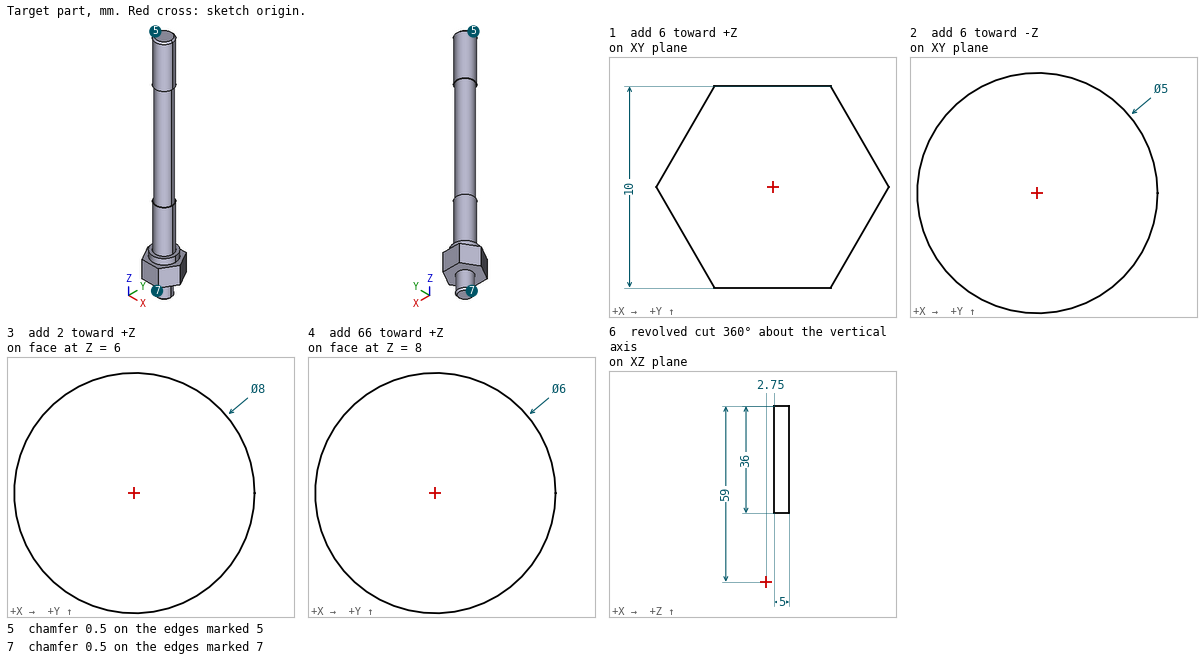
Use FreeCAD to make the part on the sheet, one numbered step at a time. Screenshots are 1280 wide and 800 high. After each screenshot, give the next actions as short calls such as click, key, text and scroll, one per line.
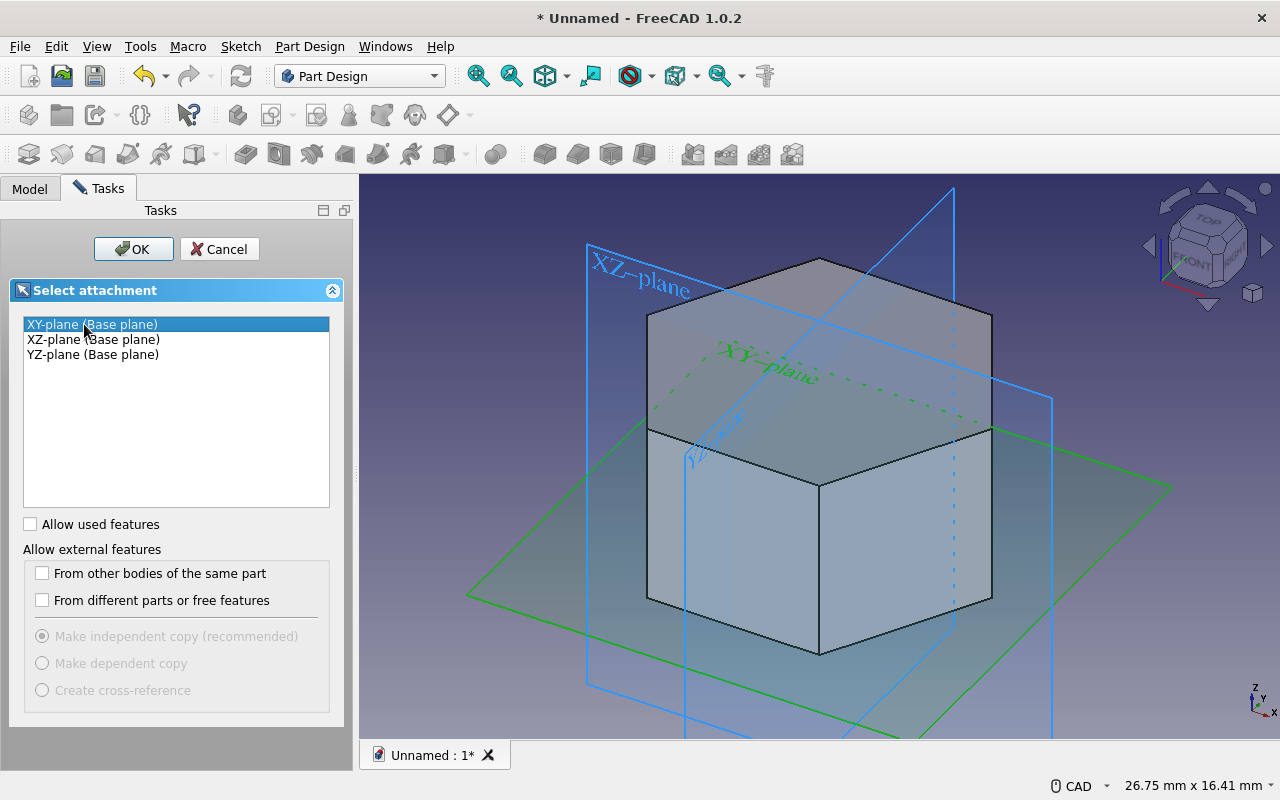
click(134, 249)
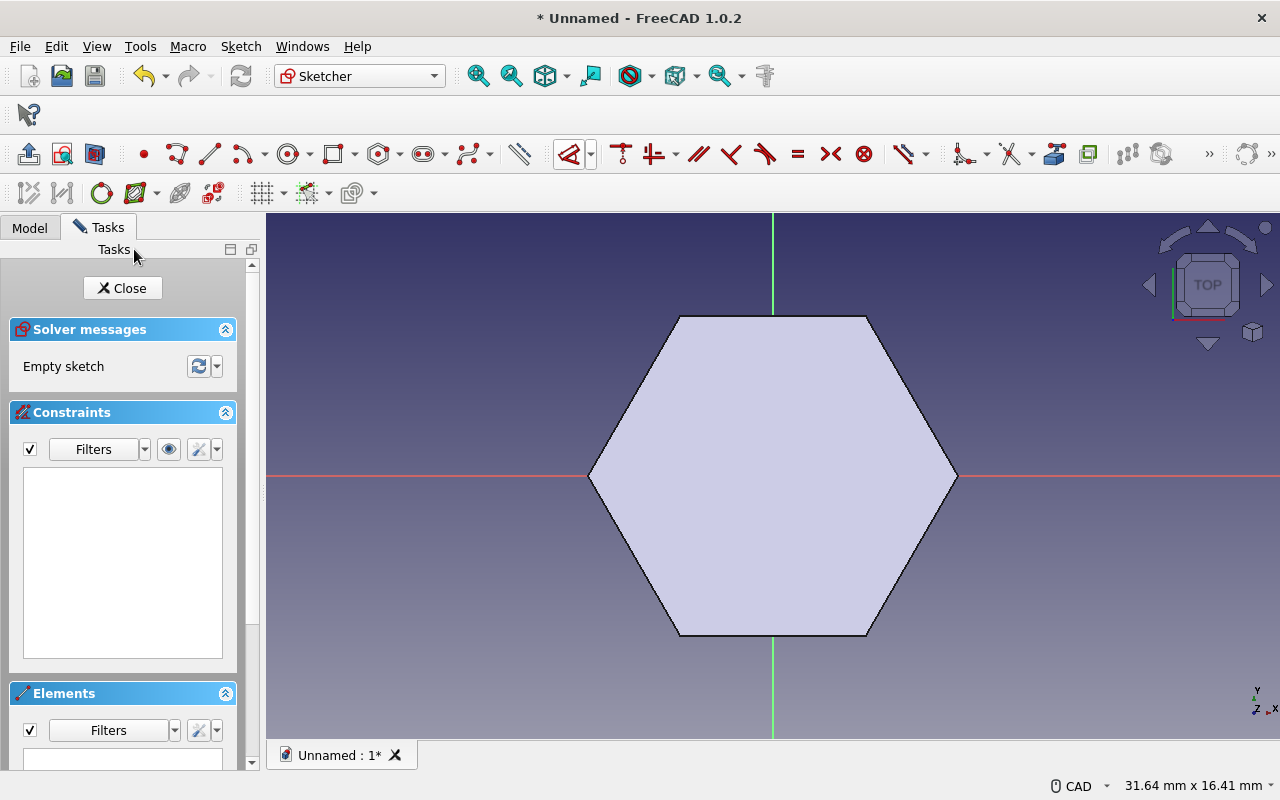
click(95, 154)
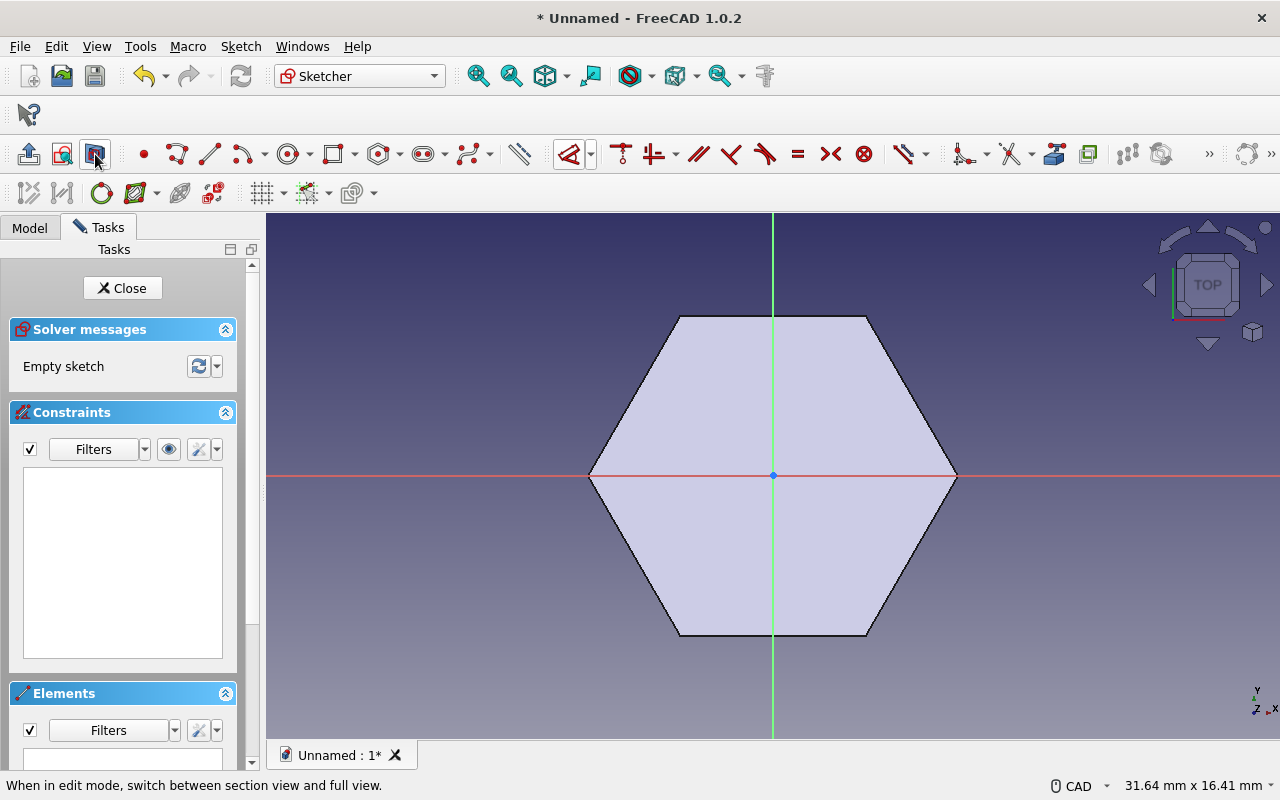
scroll(829, 476, up, 4)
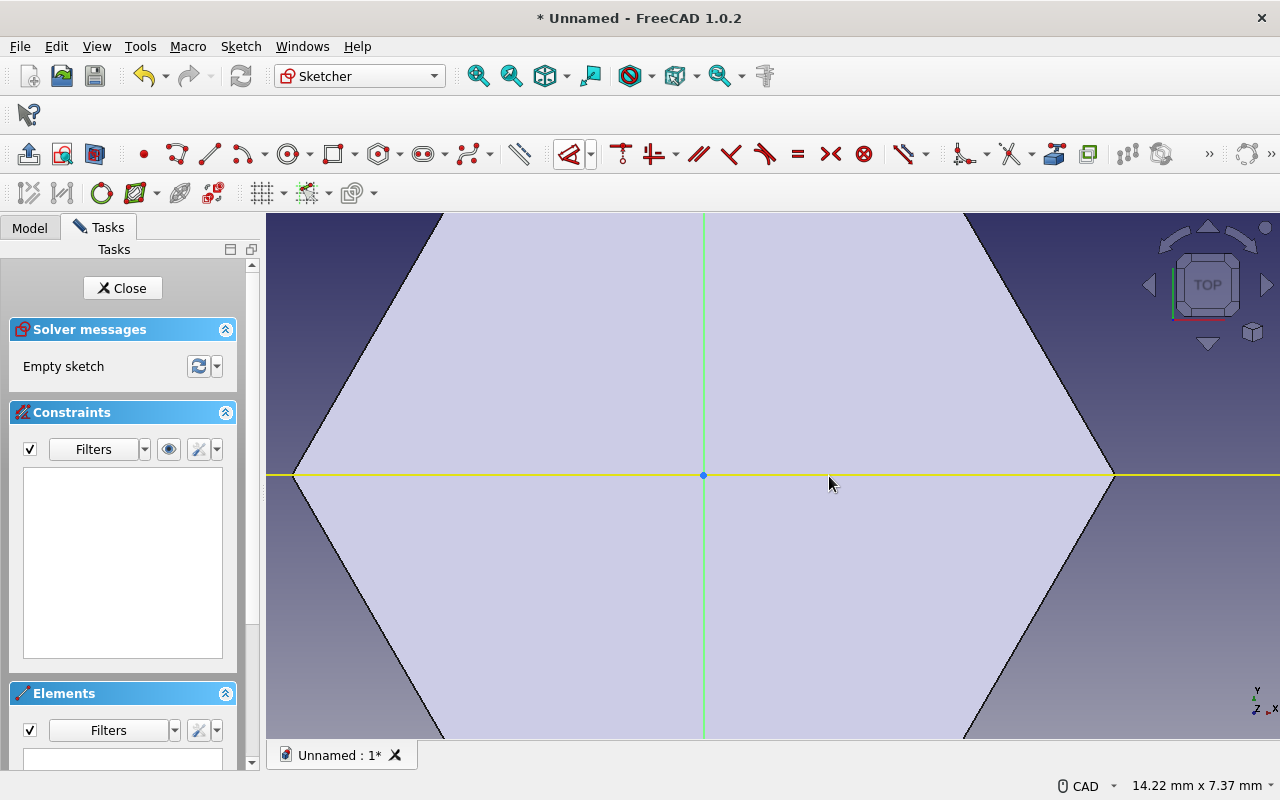
click(288, 154)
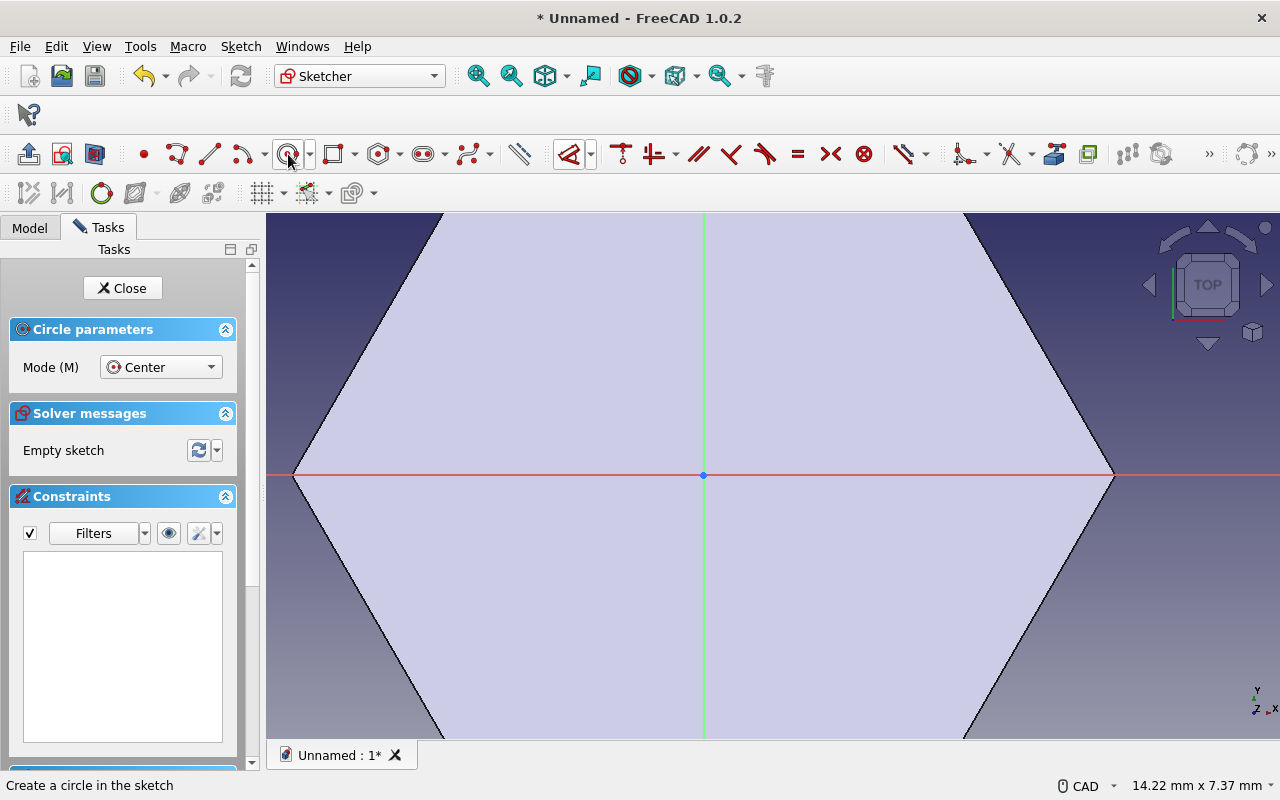
click(704, 475)
click(830, 349)
key(Escape)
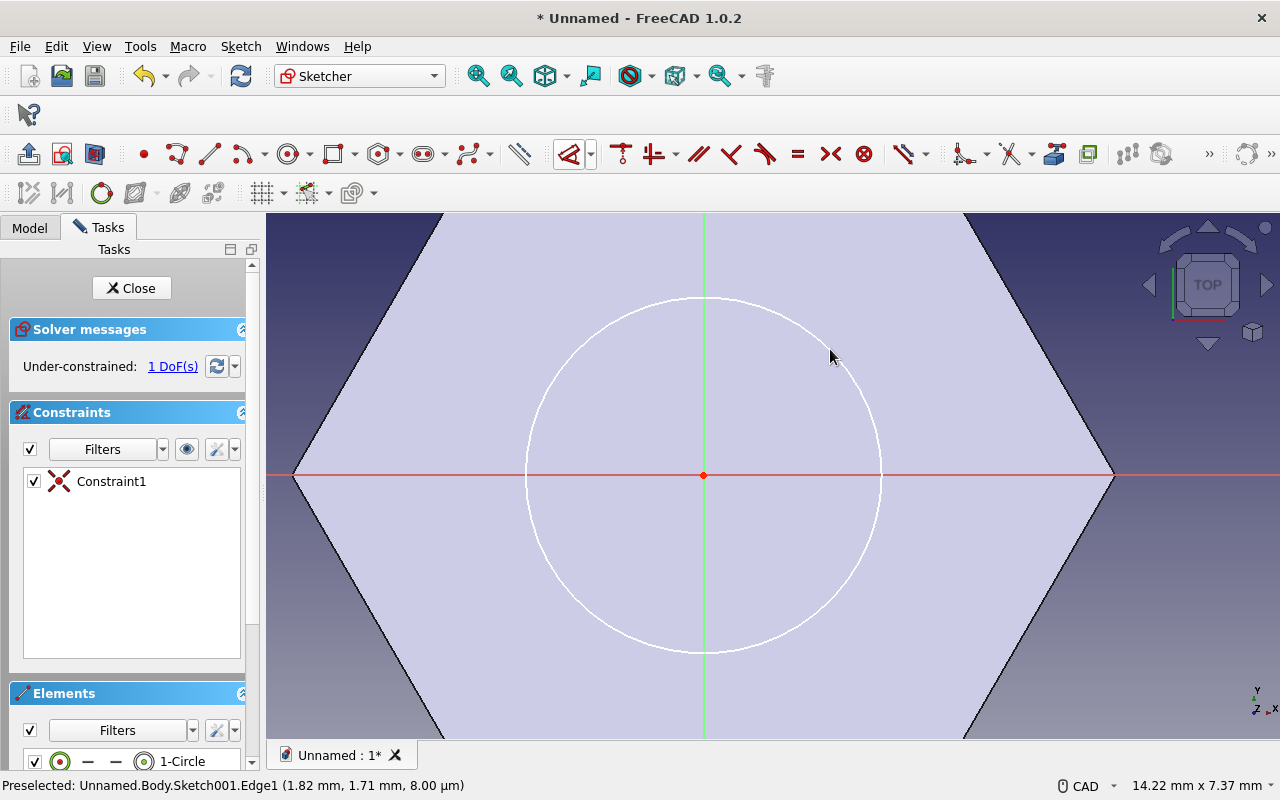
click(829, 349)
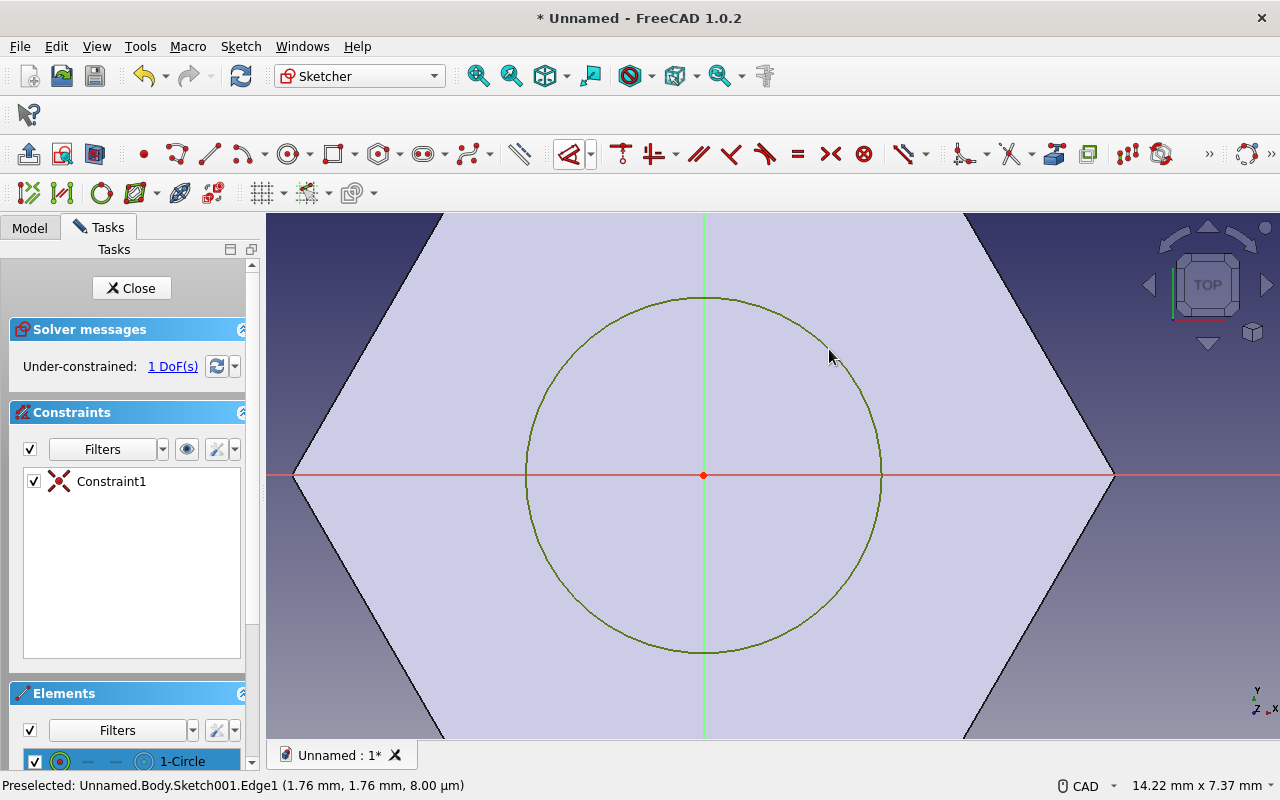
key(k)
key(o)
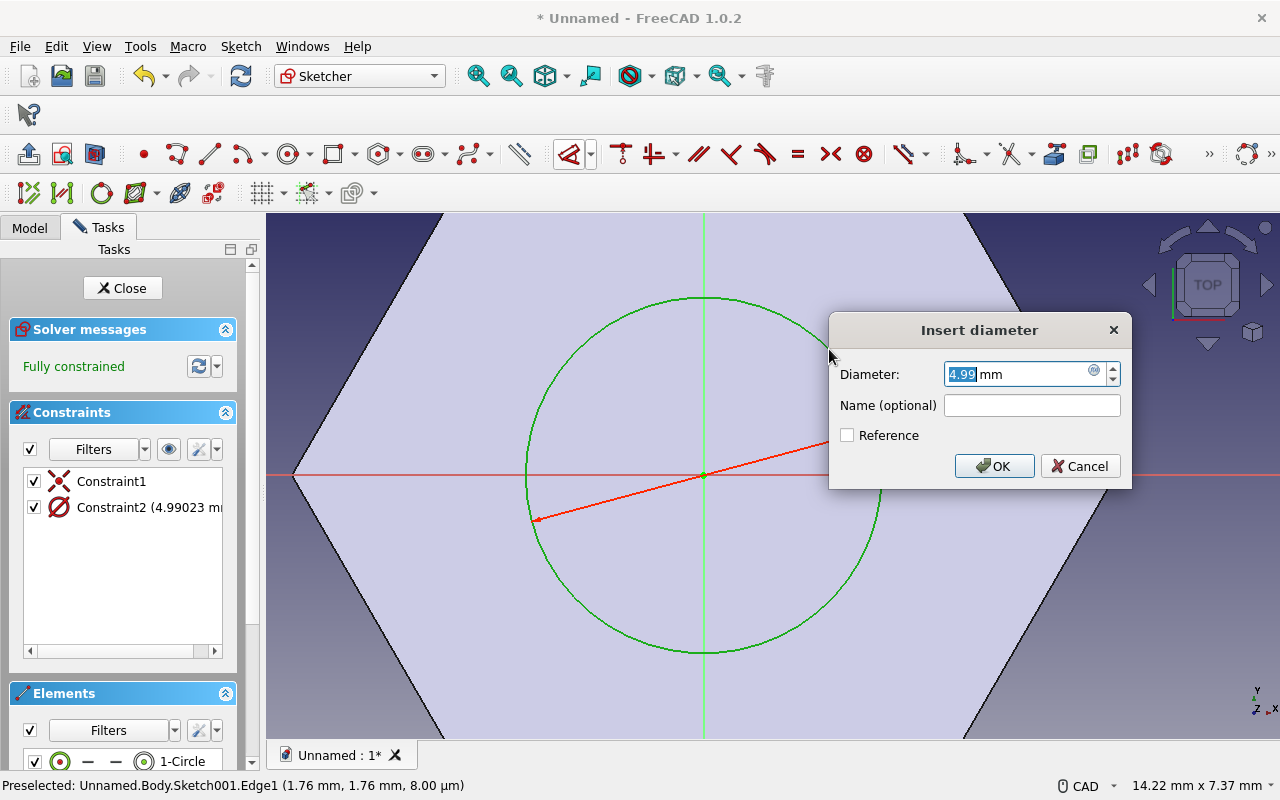
text(5)
key(Return)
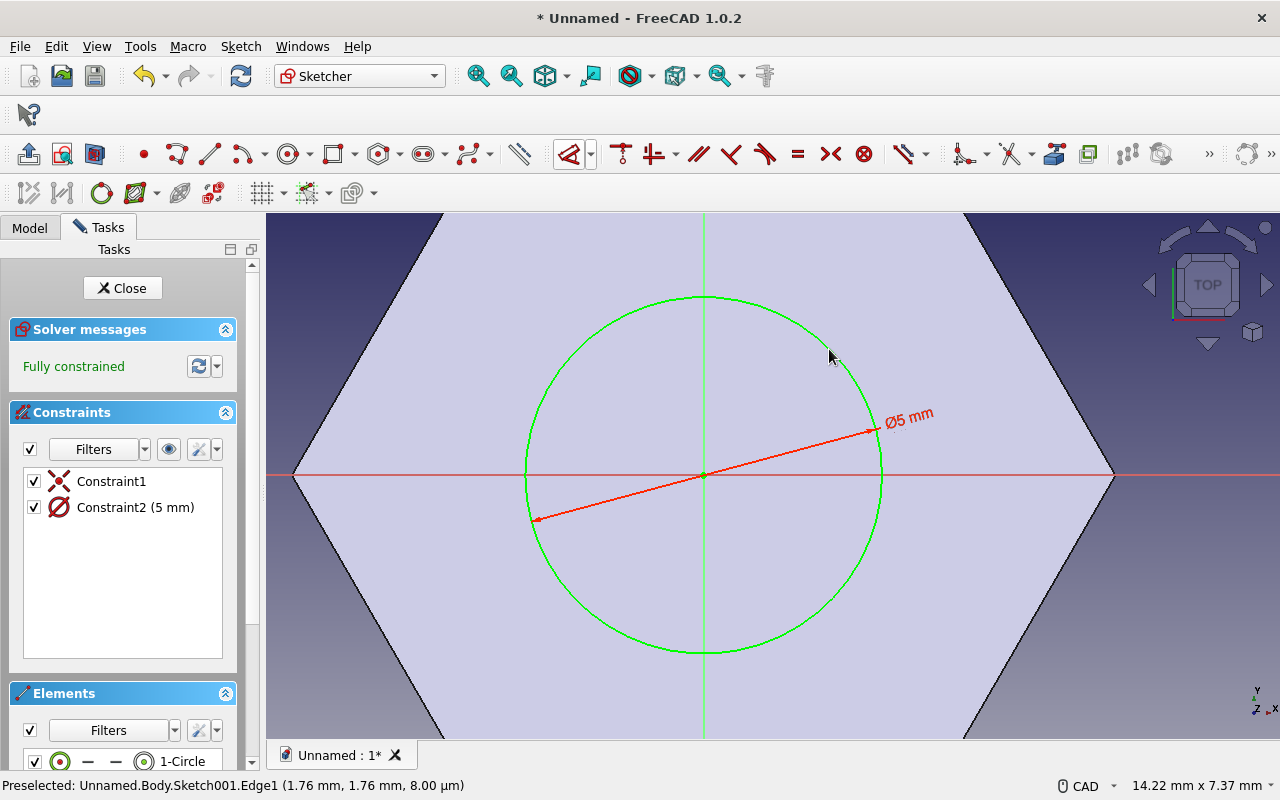
click(123, 288)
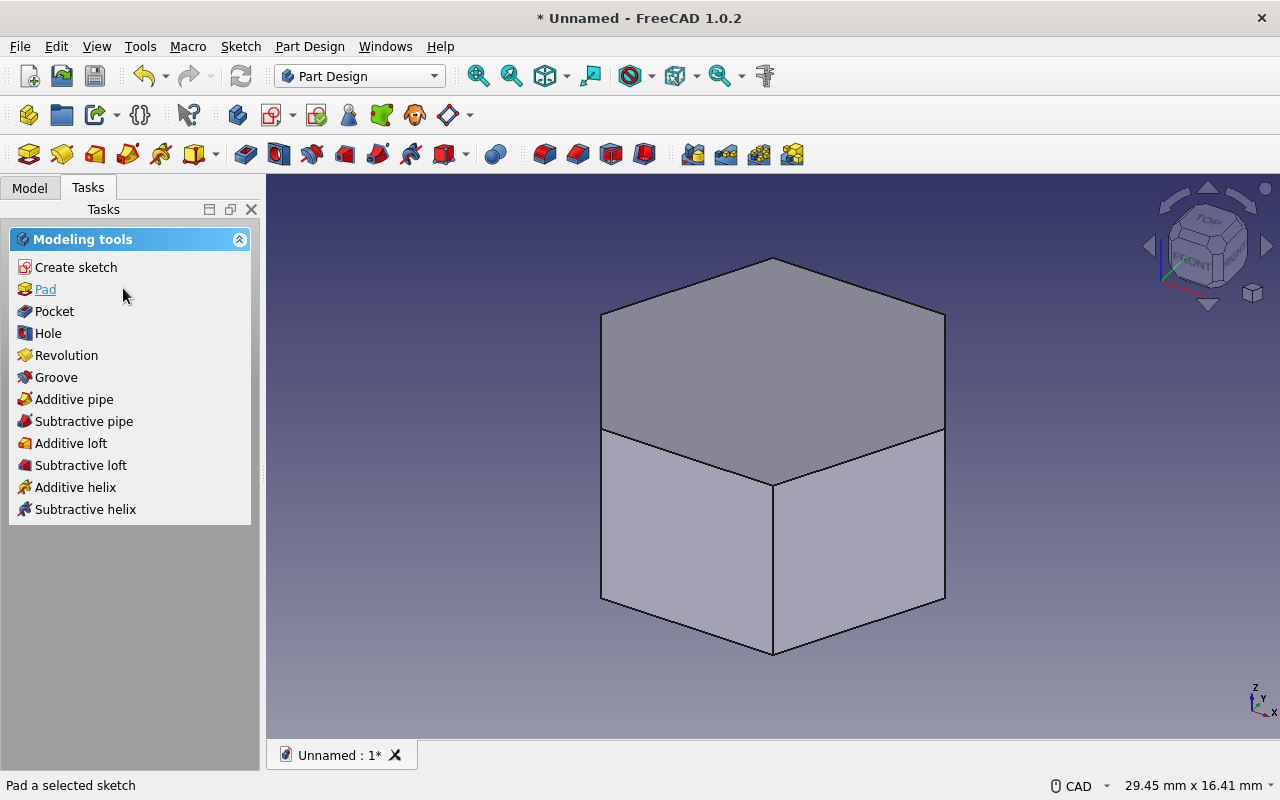
click(29, 154)